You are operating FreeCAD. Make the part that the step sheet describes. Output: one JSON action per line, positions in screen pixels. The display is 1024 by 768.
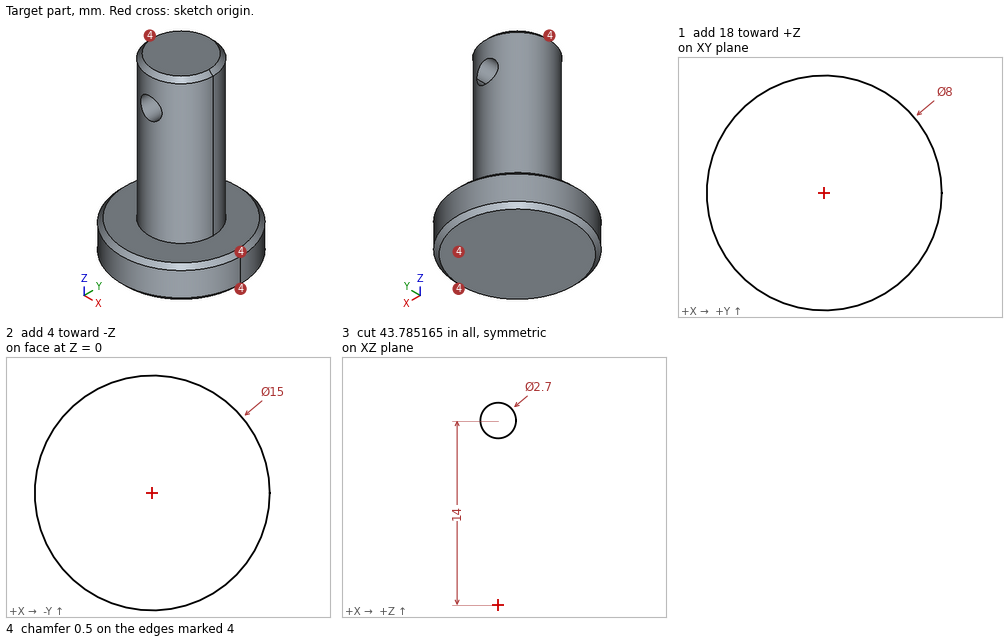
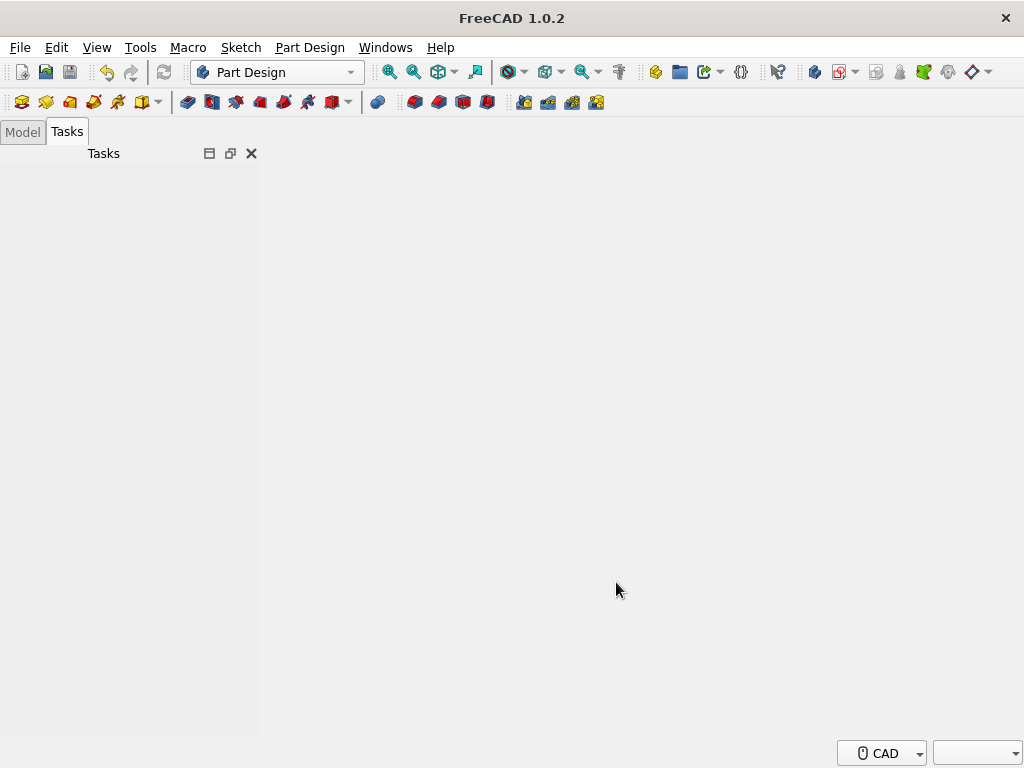
{"action": "left_click", "coordinate": [22, 72]}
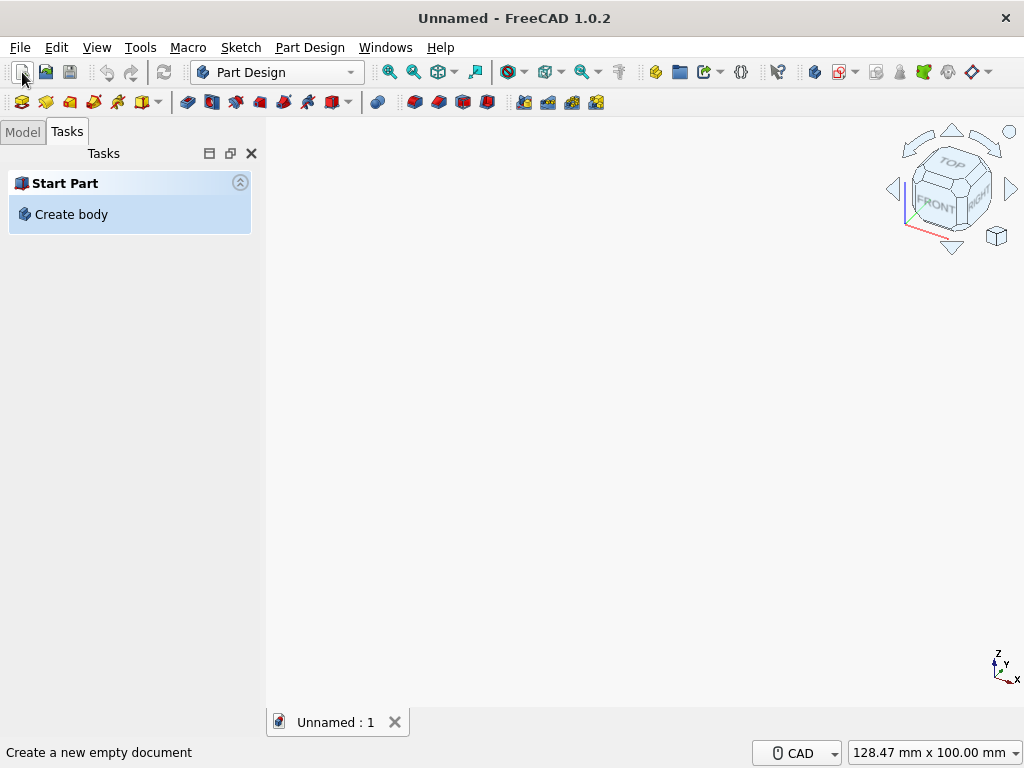
{"action": "left_click", "coordinate": [840, 72]}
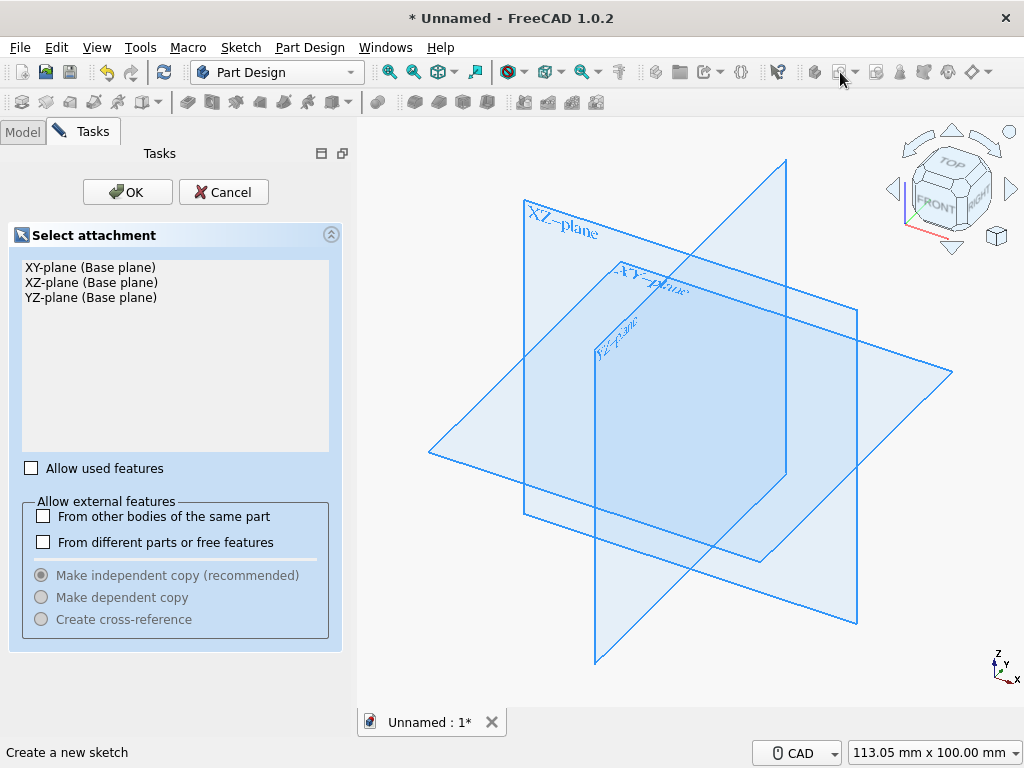
{"action": "left_click", "coordinate": [82, 268]}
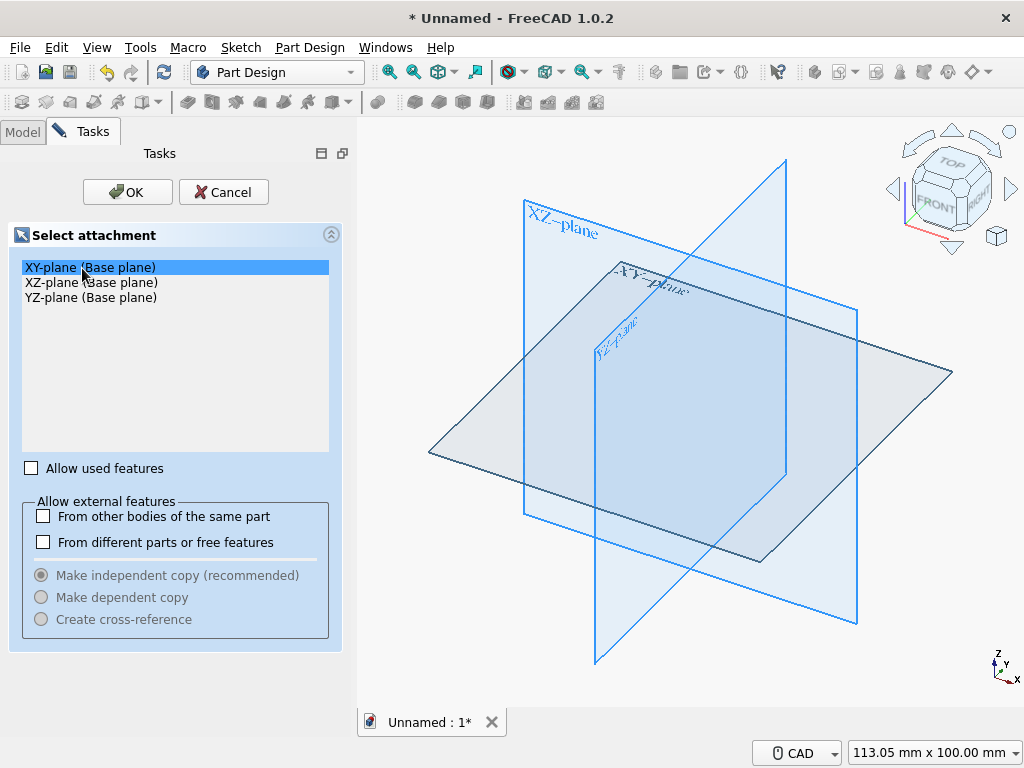
{"action": "left_click", "coordinate": [128, 192]}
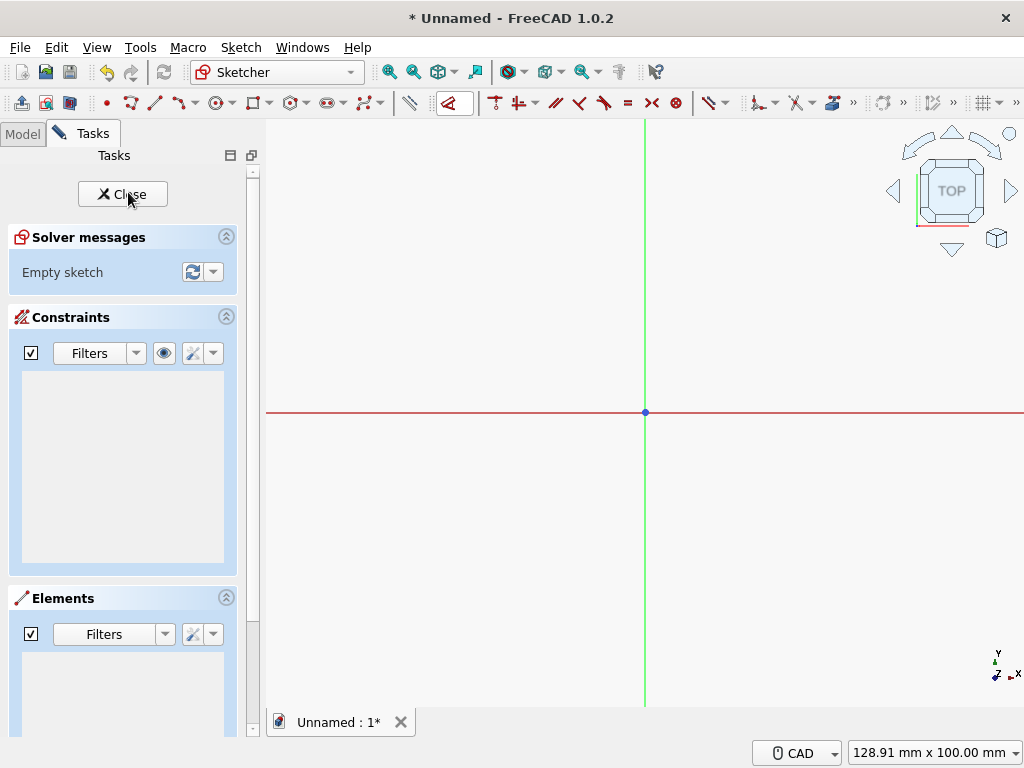
{"action": "scroll", "coordinate": [656, 413], "scroll_direction": "up", "scroll_amount": 10}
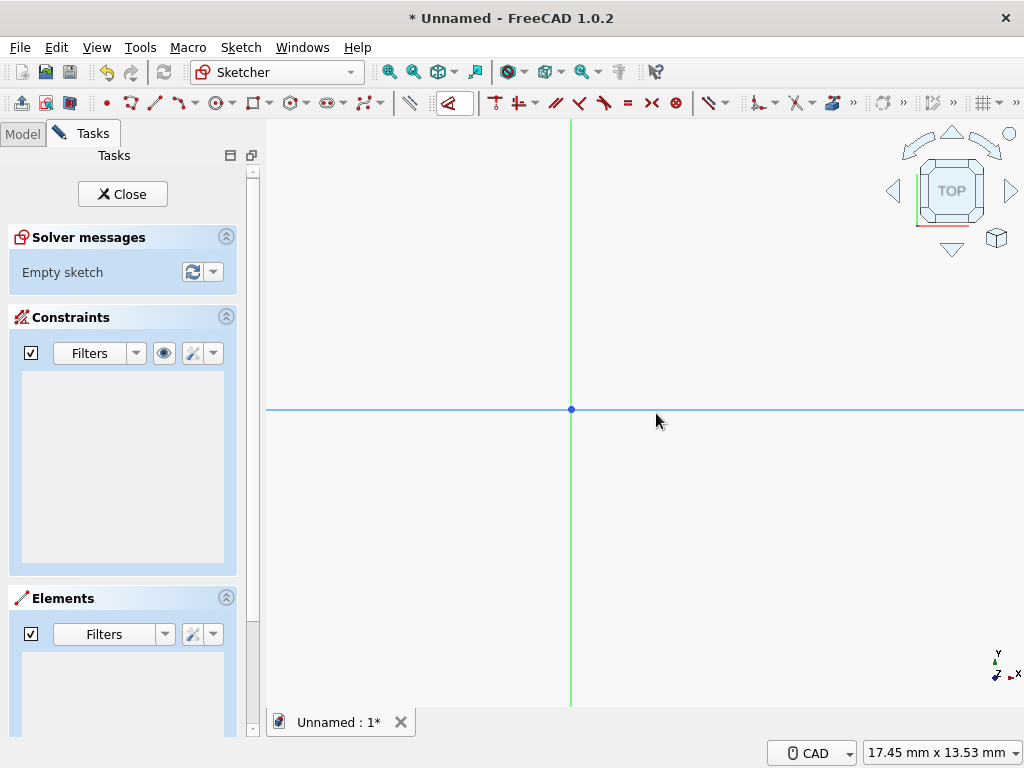
{"action": "left_click", "coordinate": [216, 104]}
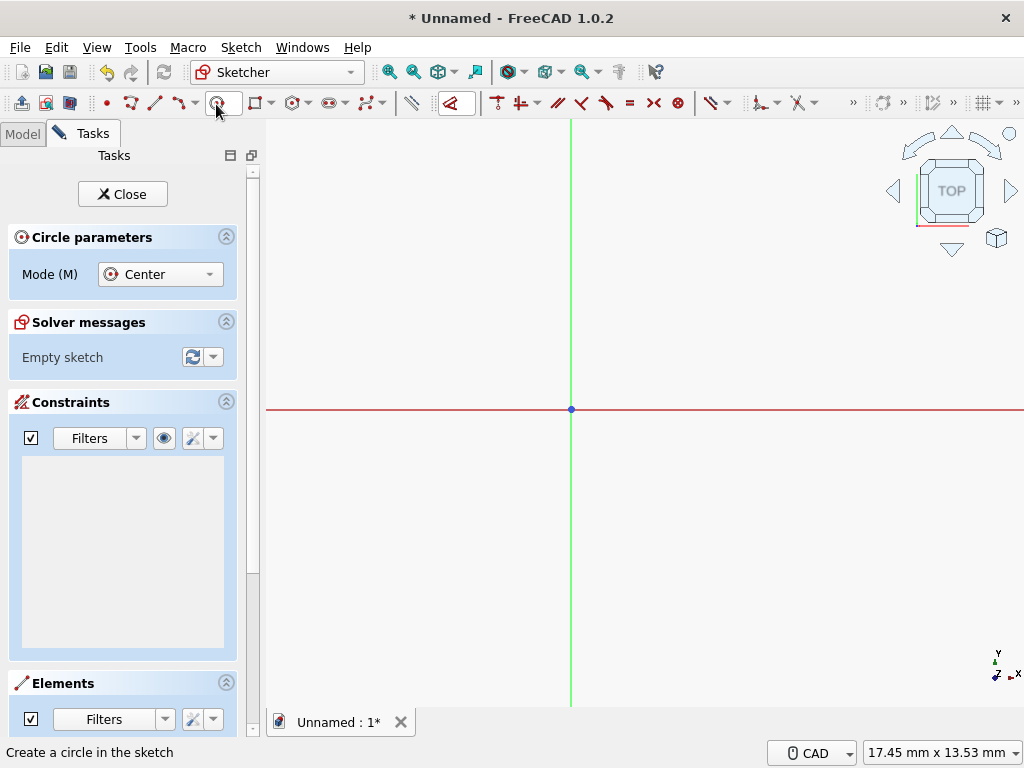
{"action": "left_click", "coordinate": [571, 410]}
{"action": "left_click", "coordinate": [694, 287]}
{"action": "key", "text": "Escape"}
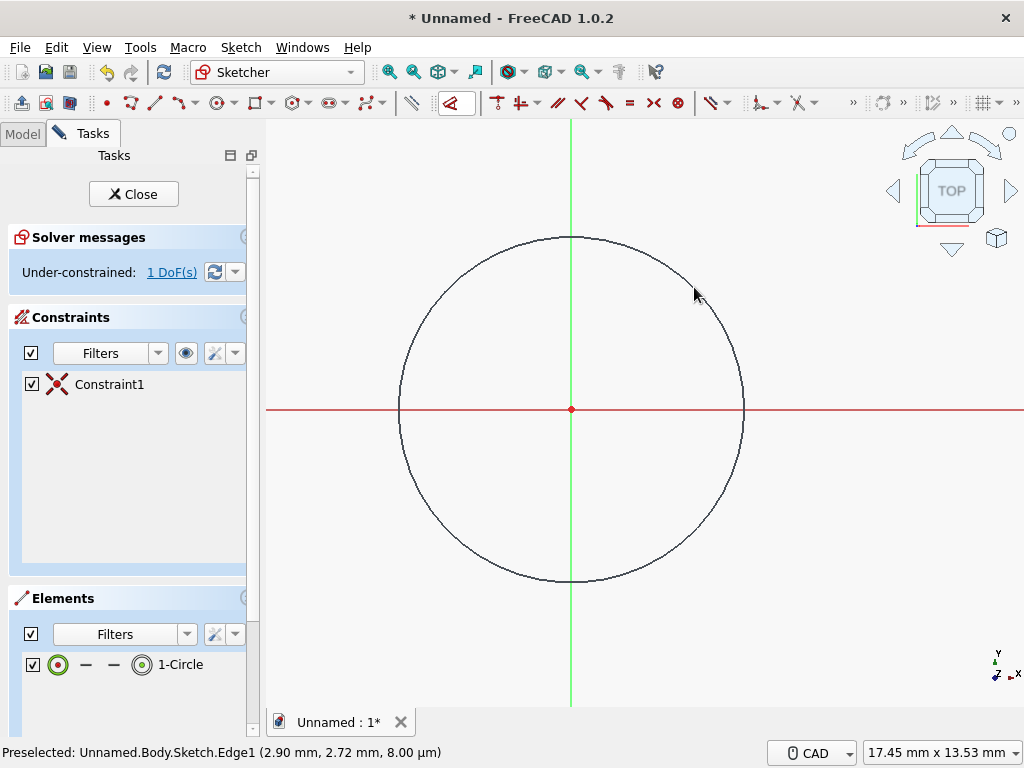
{"action": "left_click", "coordinate": [450, 104]}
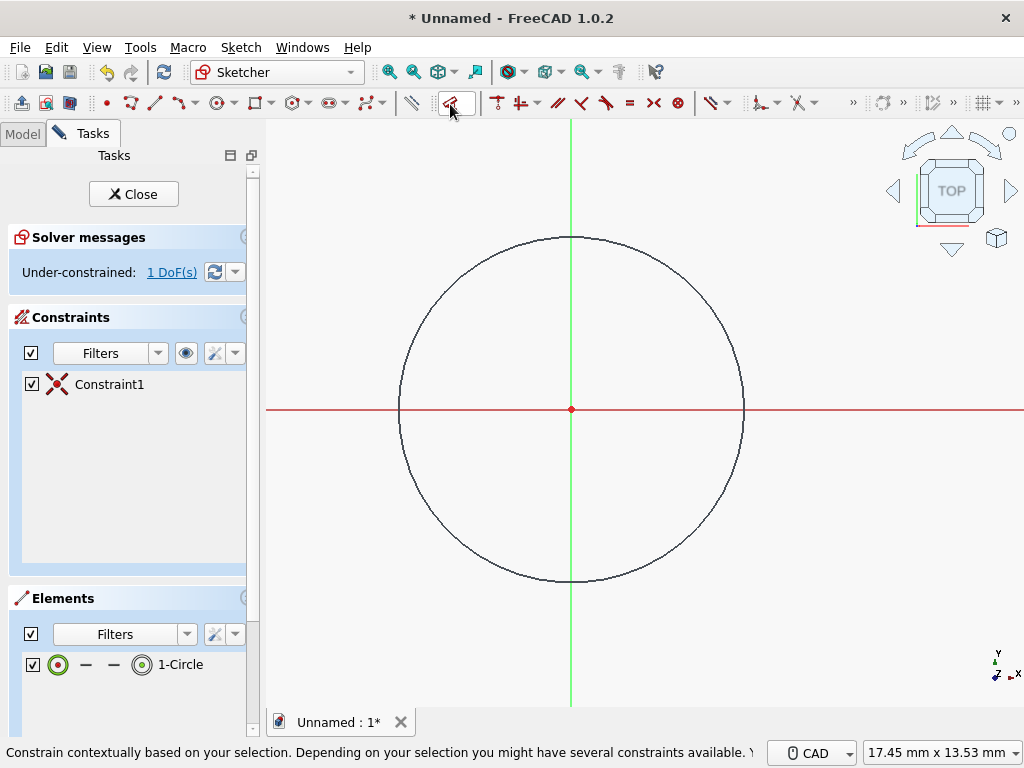
{"action": "left_click", "coordinate": [693, 287]}
{"action": "left_click", "coordinate": [716, 264]}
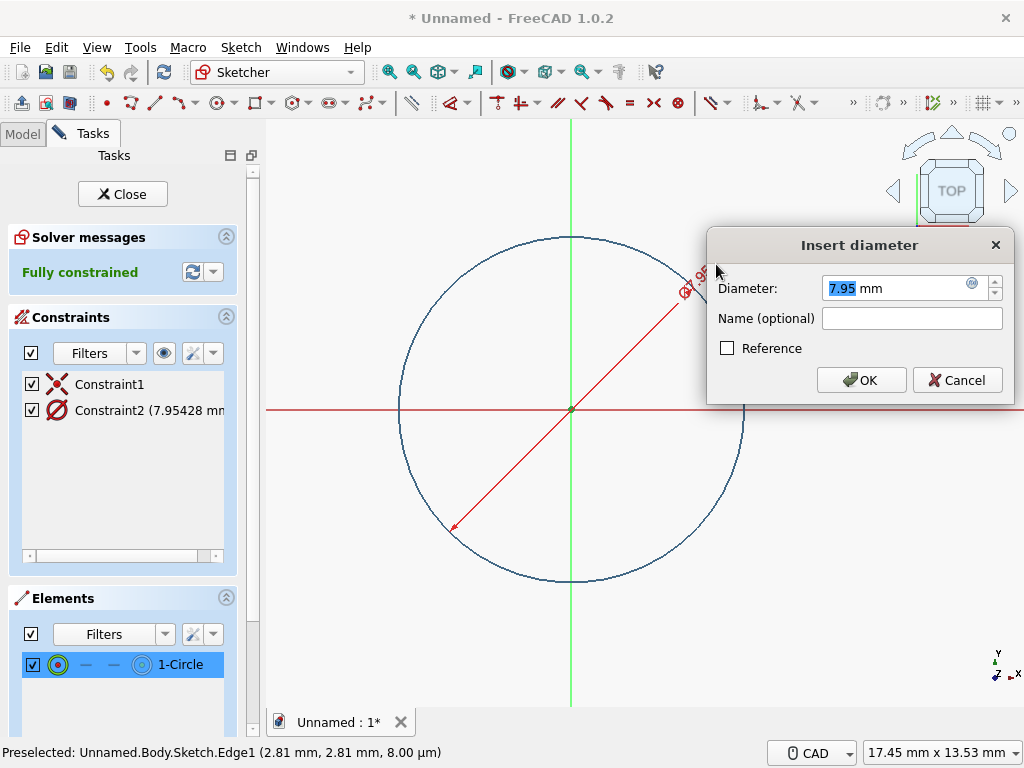
{"action": "type", "text": "8"}
{"action": "key", "text": "Return"}
{"action": "key", "text": "Escape"}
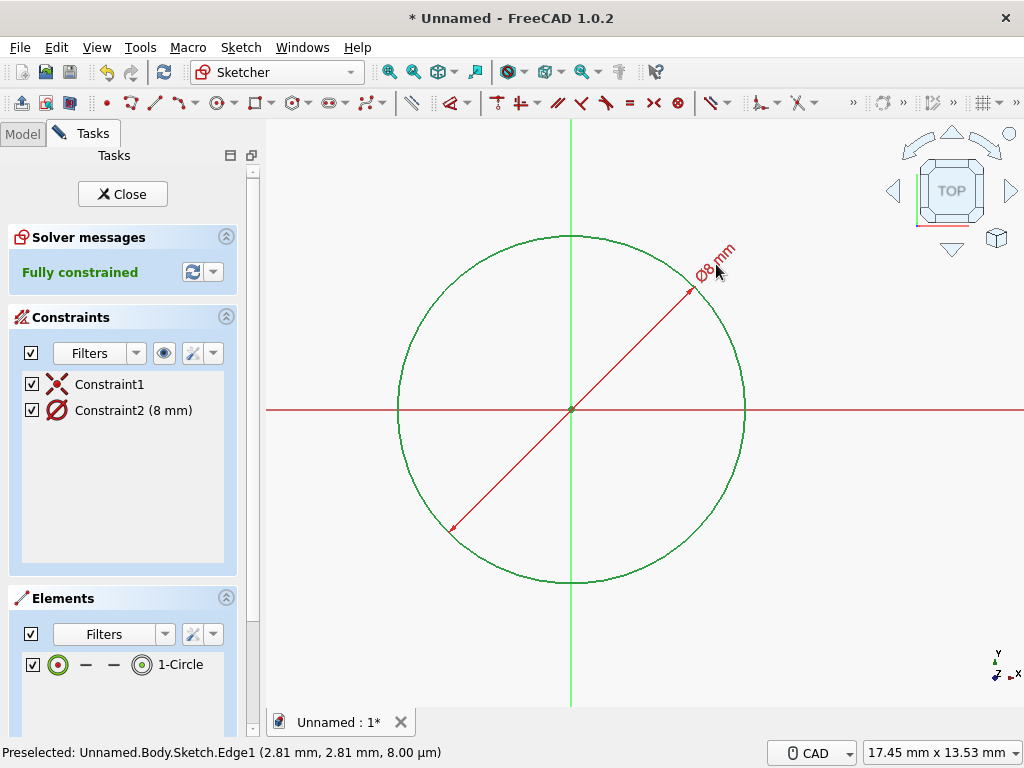
{"action": "left_click", "coordinate": [123, 194]}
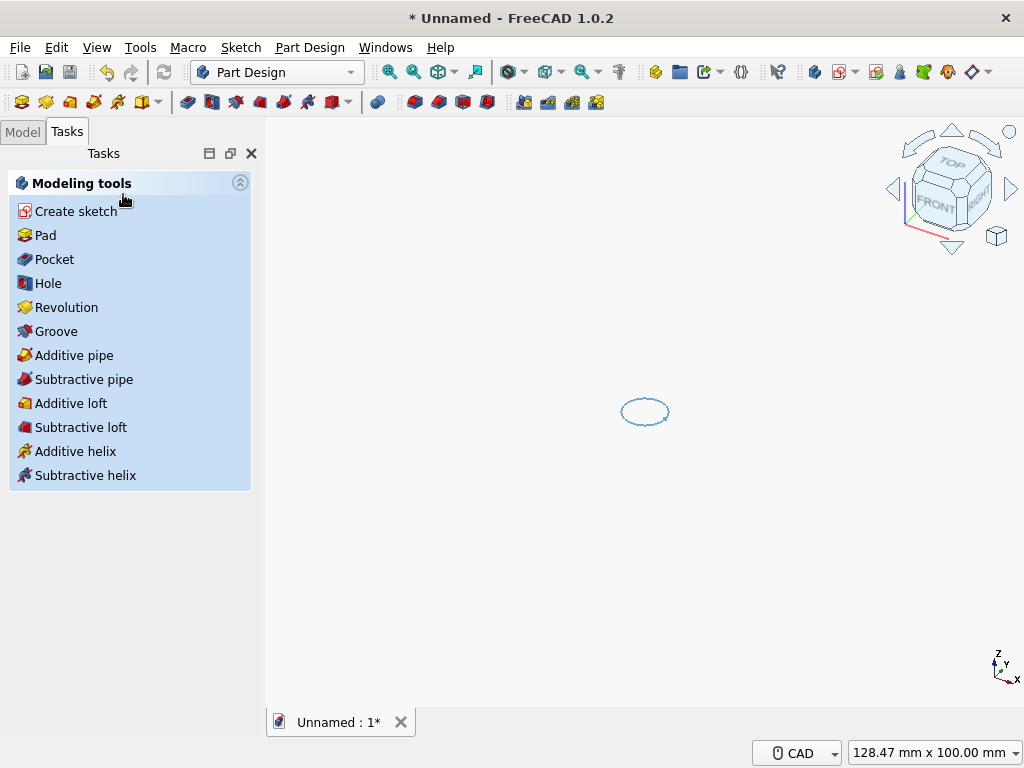
{"action": "left_click", "coordinate": [22, 102]}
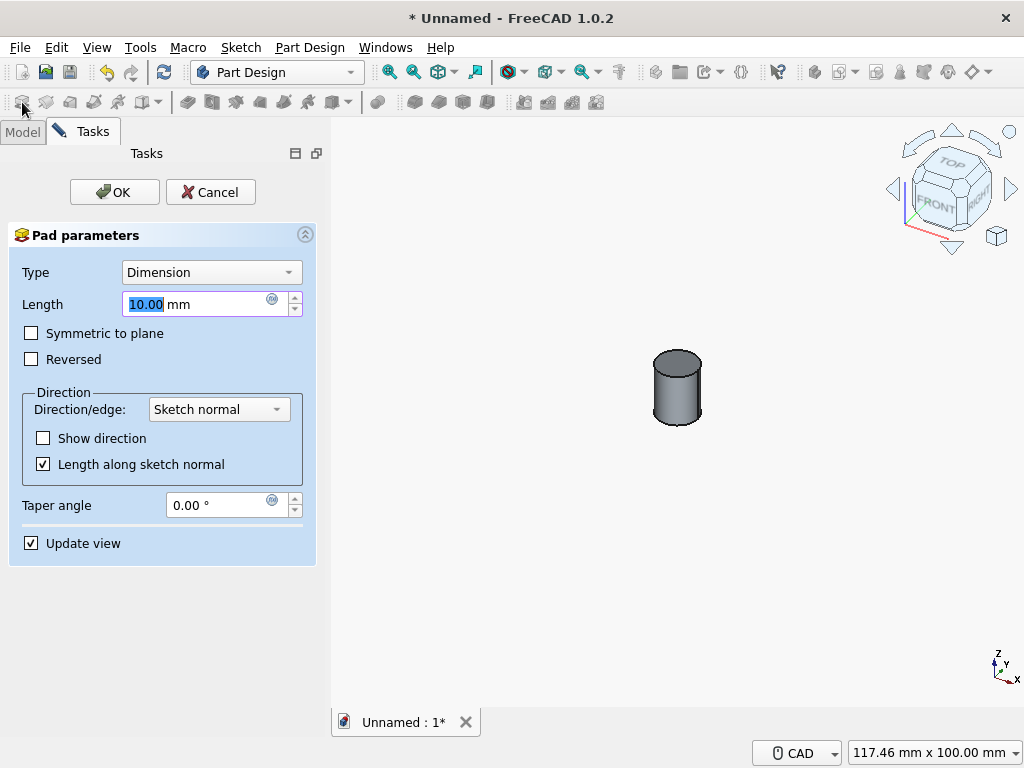
{"action": "type", "text": "18"}
{"action": "key", "text": "Tab"}